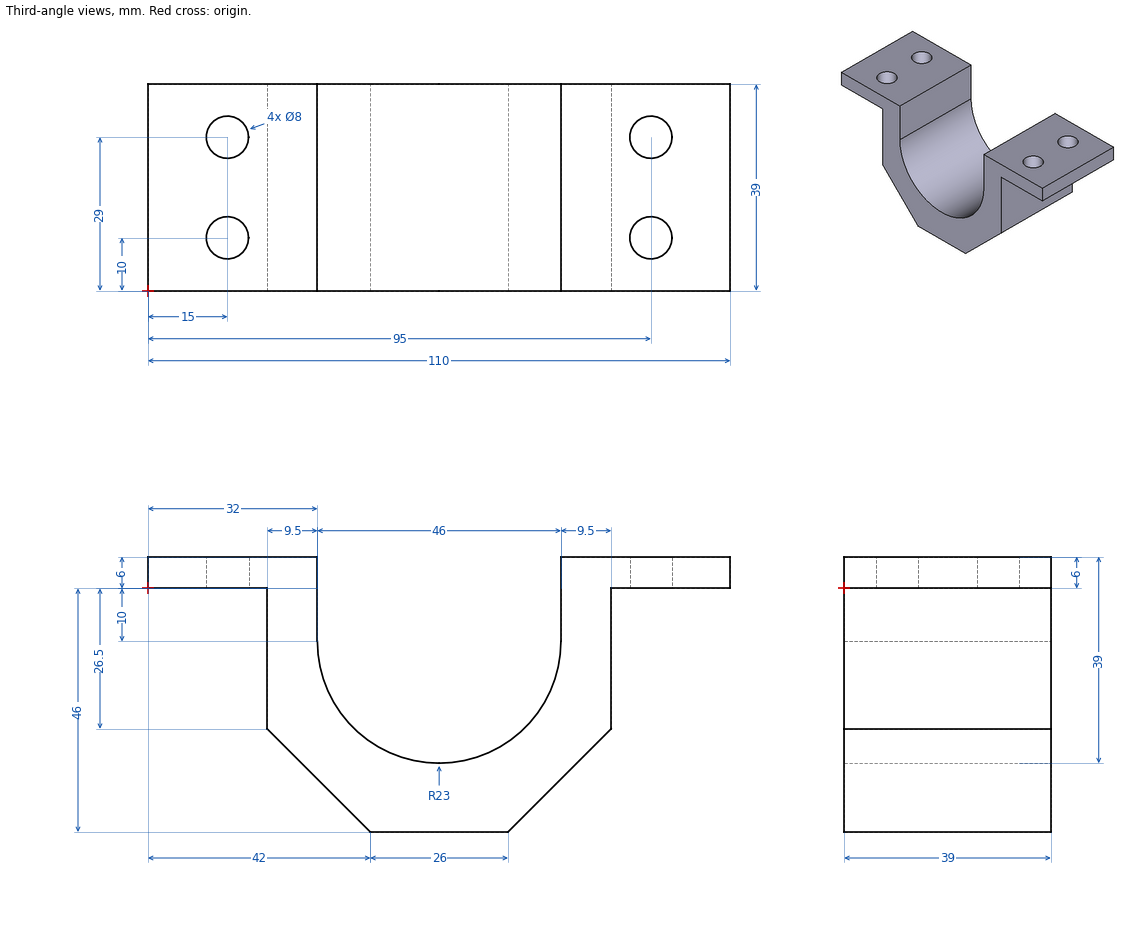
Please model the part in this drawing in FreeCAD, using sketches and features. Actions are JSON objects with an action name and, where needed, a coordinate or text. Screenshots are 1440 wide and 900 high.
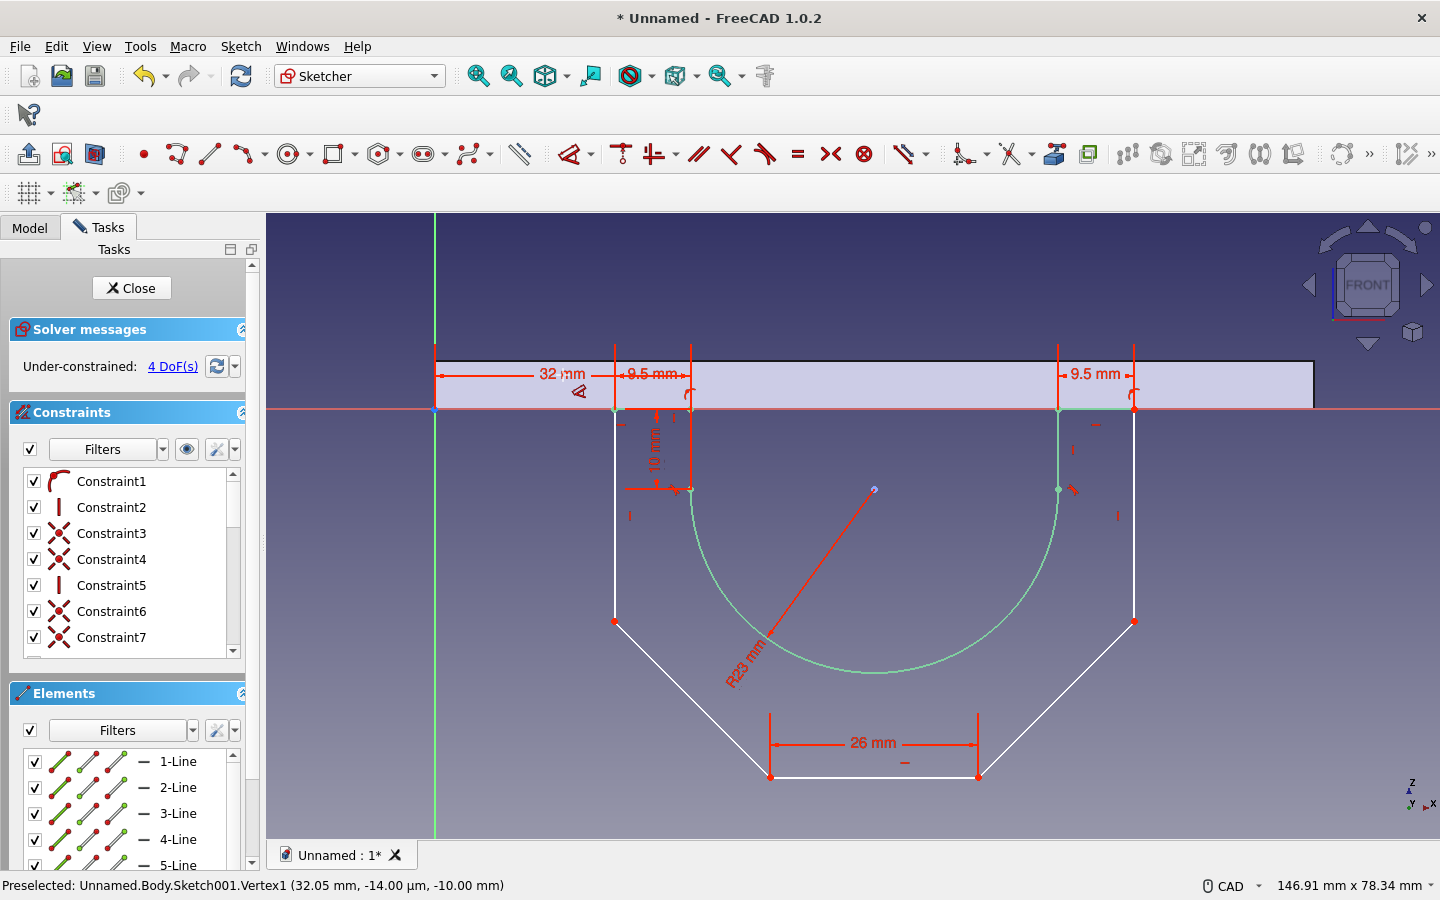
{"action": "left_click", "coordinate": [770, 778]}
{"action": "left_click", "coordinate": [485, 375]}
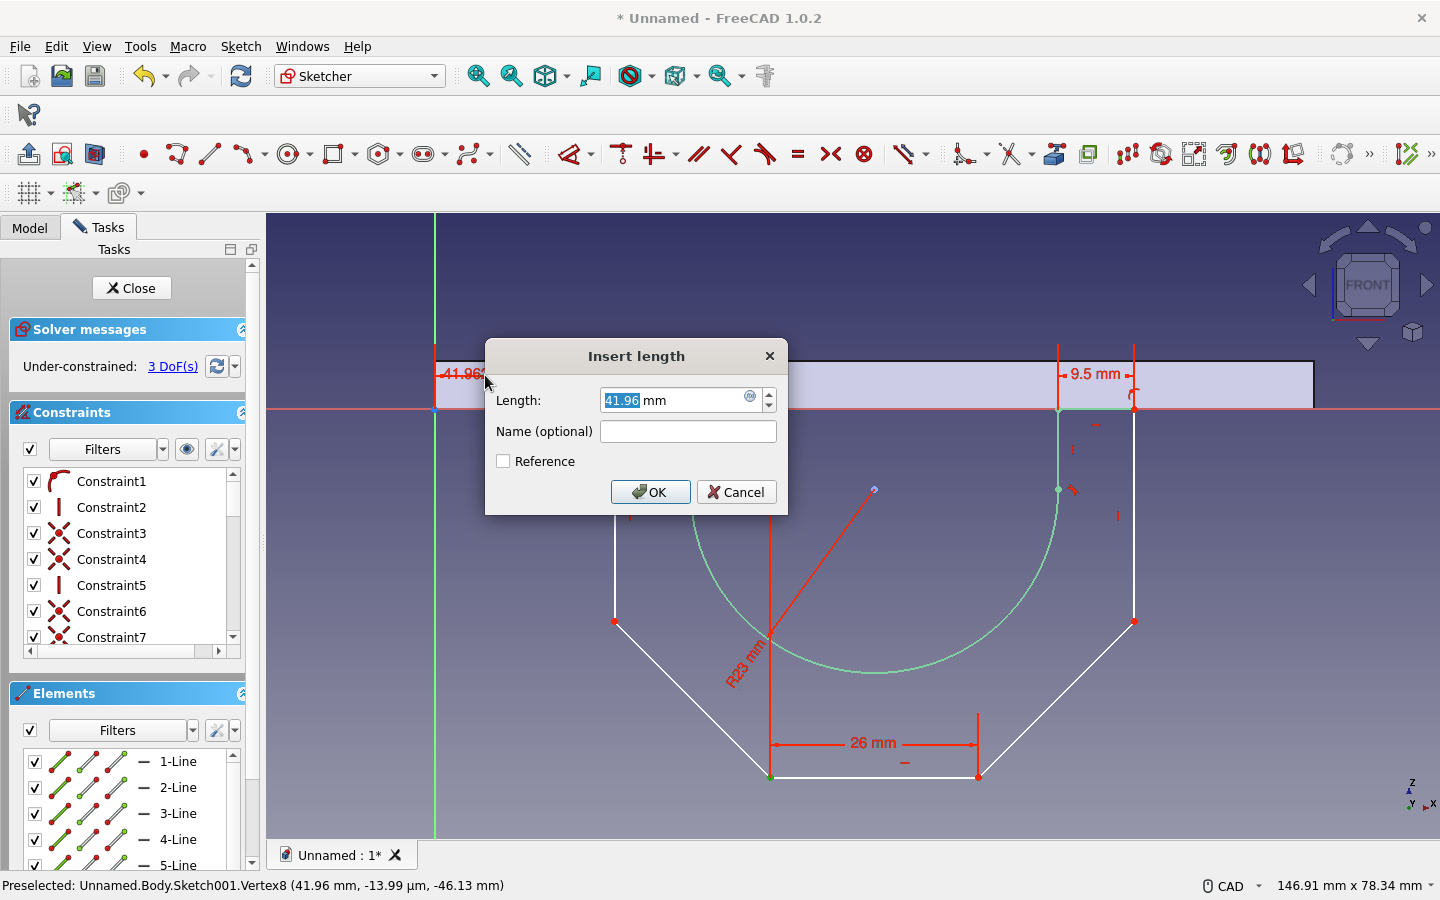
{"action": "type", "text": "42"}
{"action": "key", "text": "Return"}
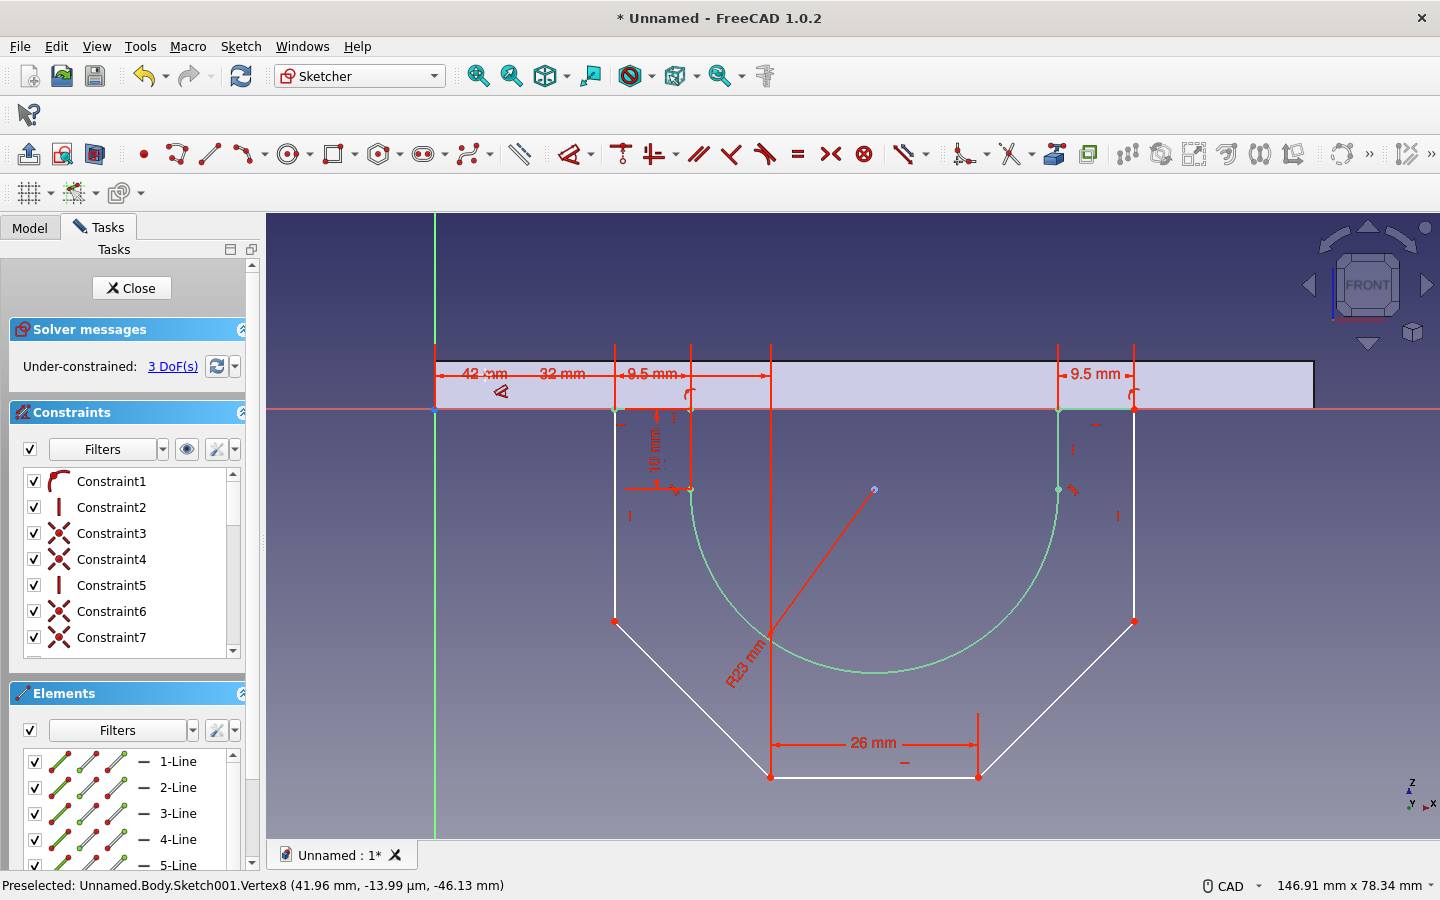
{"action": "left_click", "coordinate": [771, 778]}
{"action": "left_click", "coordinate": [401, 594]}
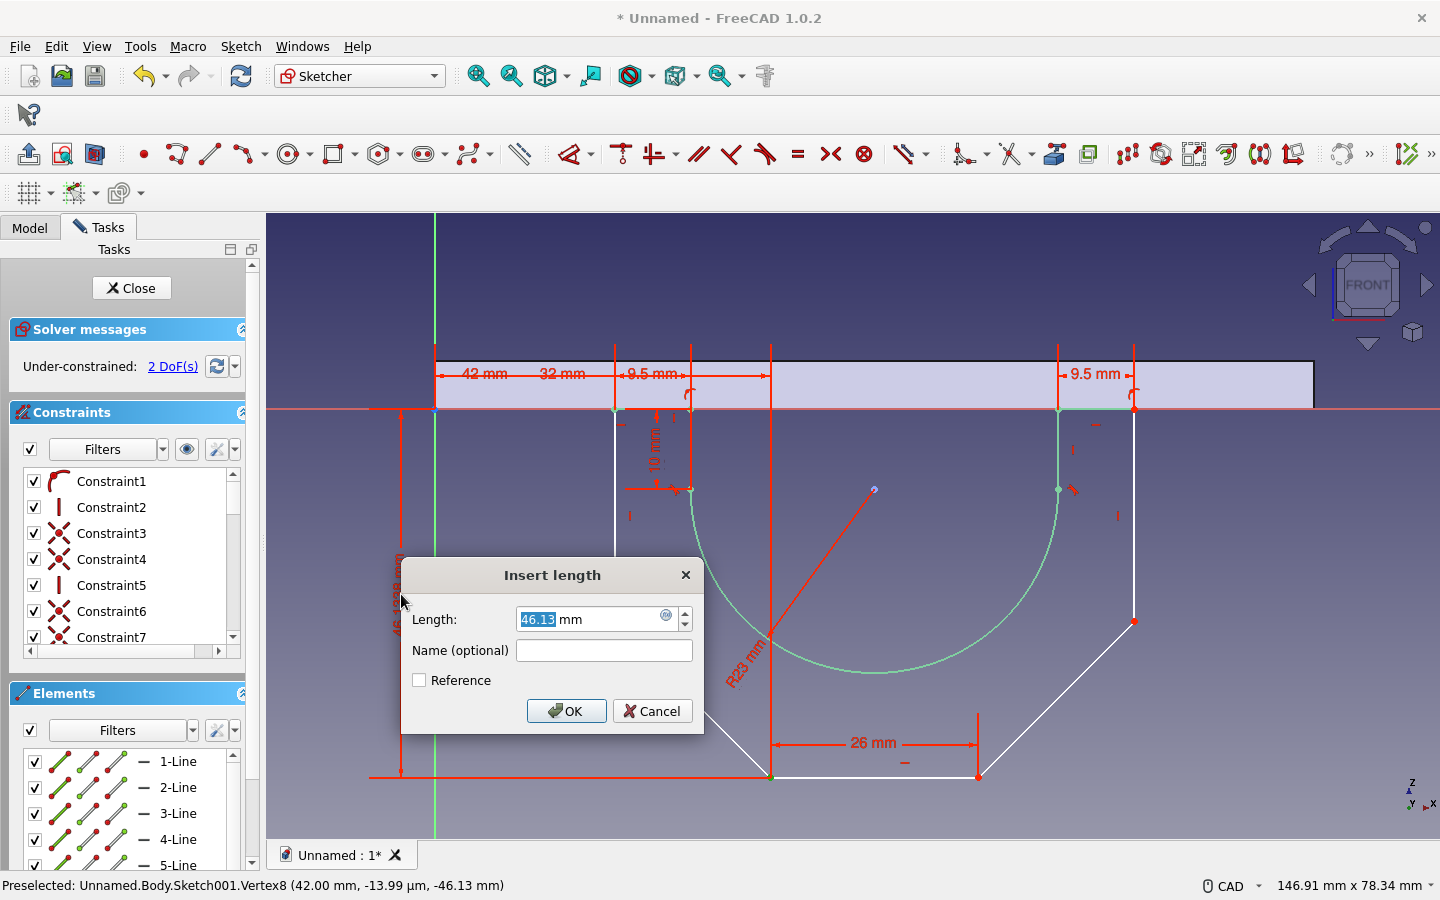
{"action": "type", "text": "46"}
{"action": "key", "text": "Return"}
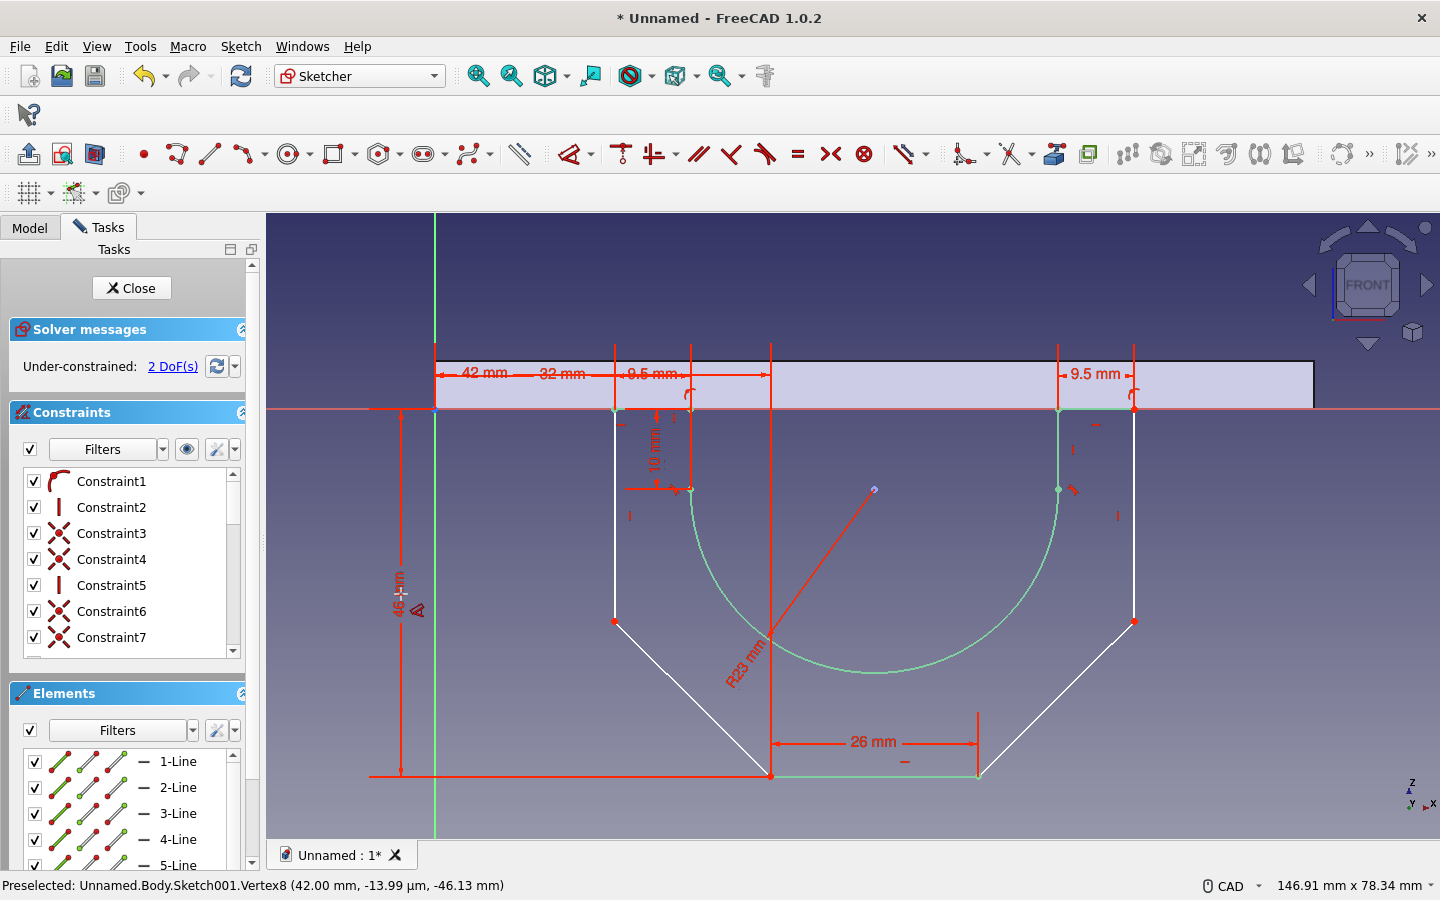
{"action": "left_click", "coordinate": [615, 473]}
{"action": "left_click", "coordinate": [581, 516]}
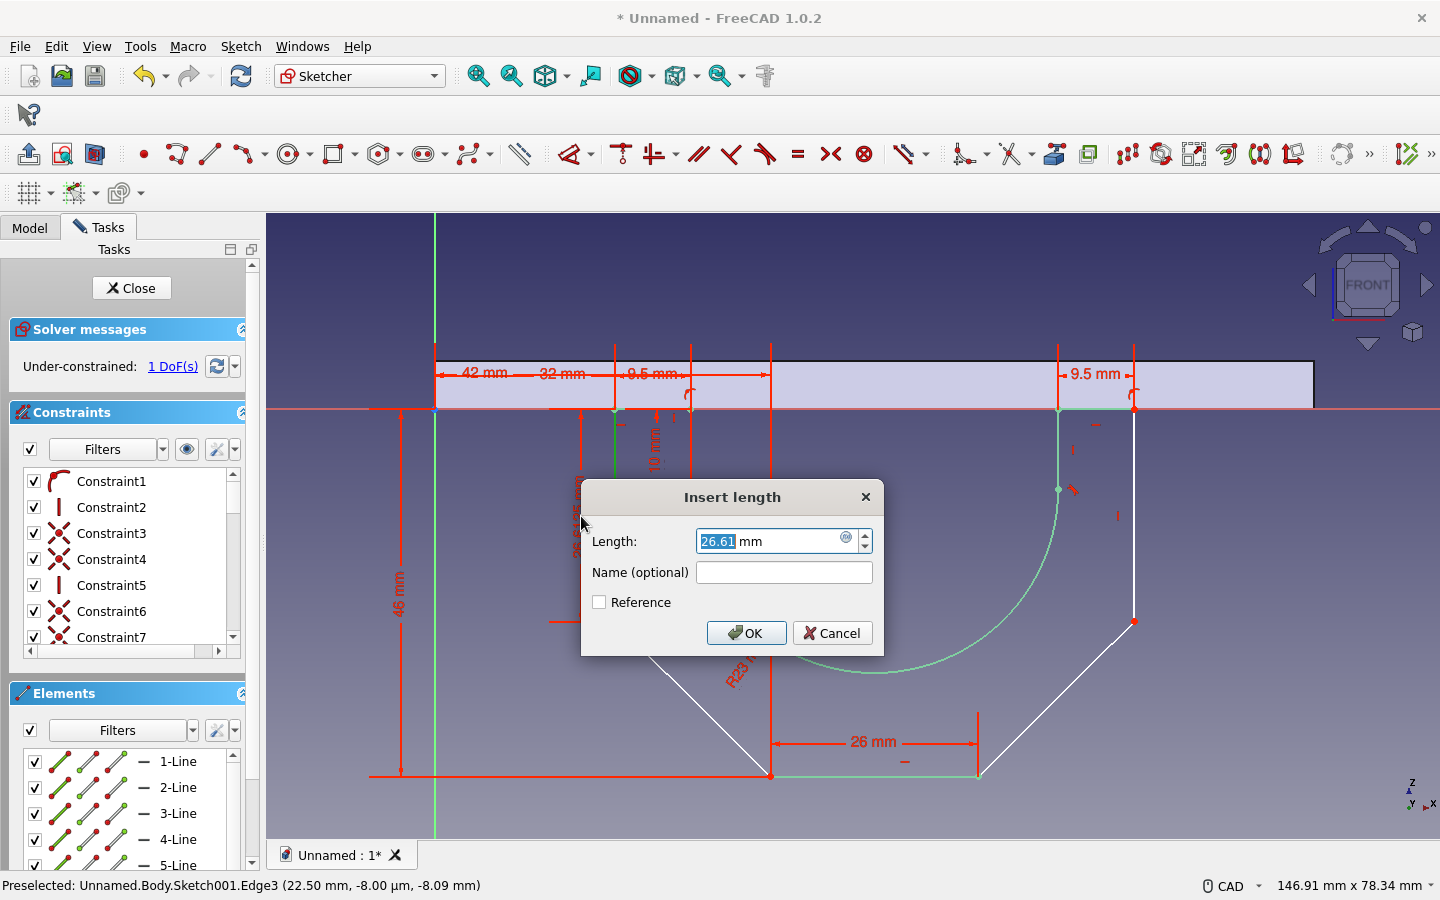
{"action": "type", "text": "26.5"}
{"action": "key", "text": "Return"}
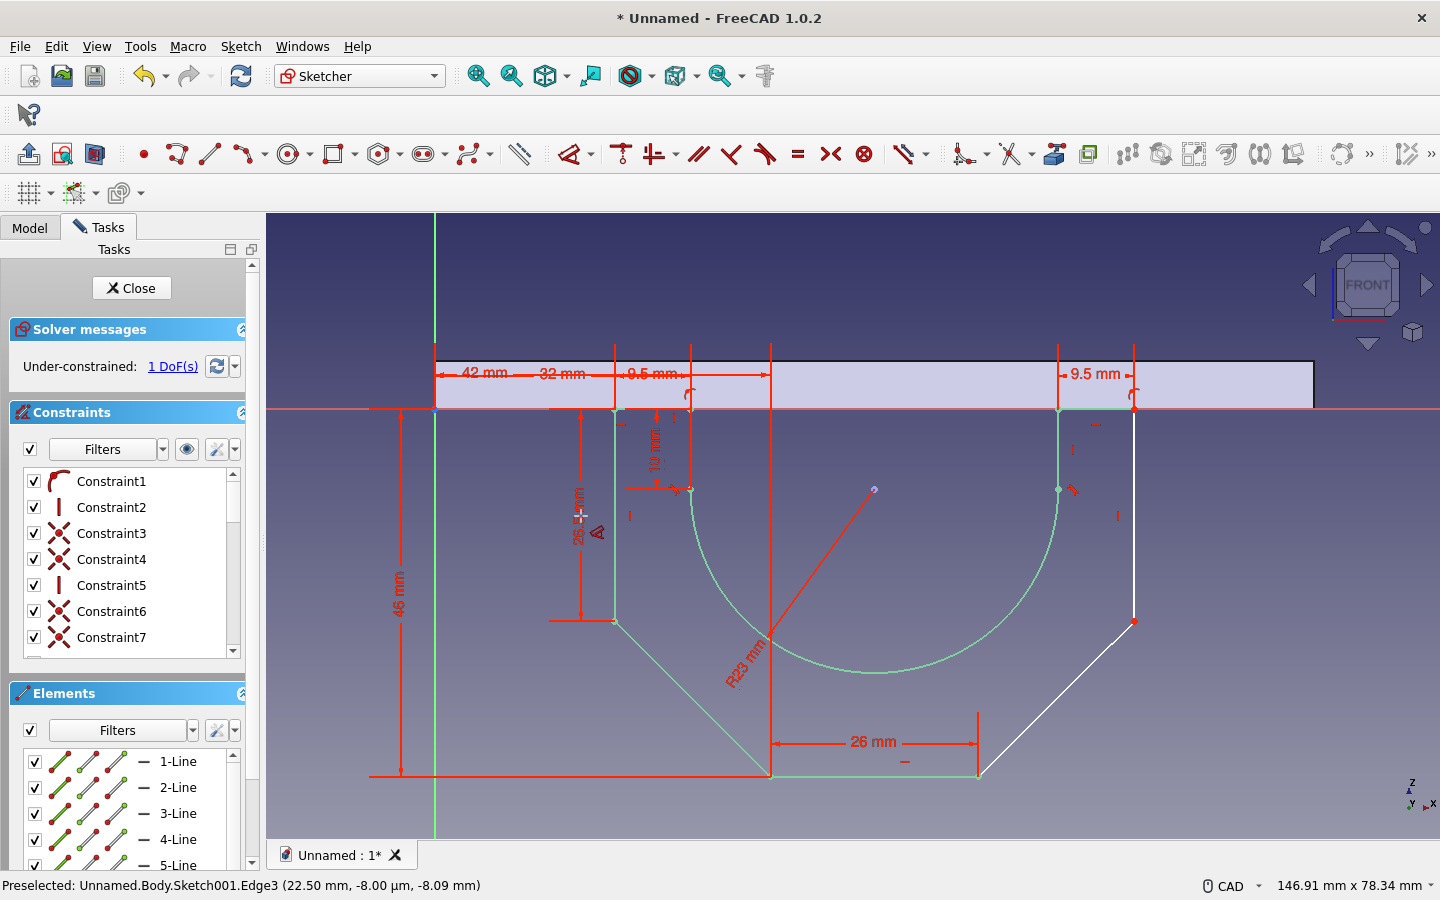
{"action": "left_click", "coordinate": [1134, 558]}
{"action": "left_click", "coordinate": [1168, 516]}